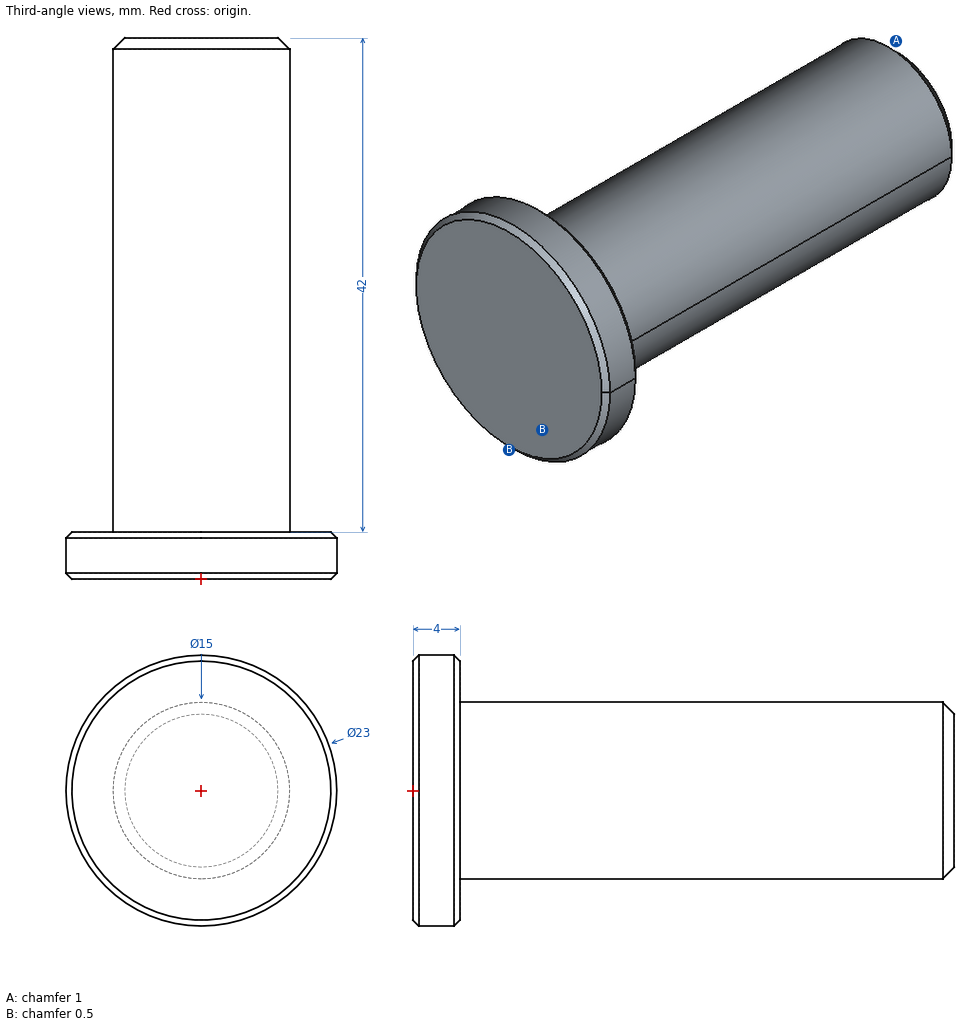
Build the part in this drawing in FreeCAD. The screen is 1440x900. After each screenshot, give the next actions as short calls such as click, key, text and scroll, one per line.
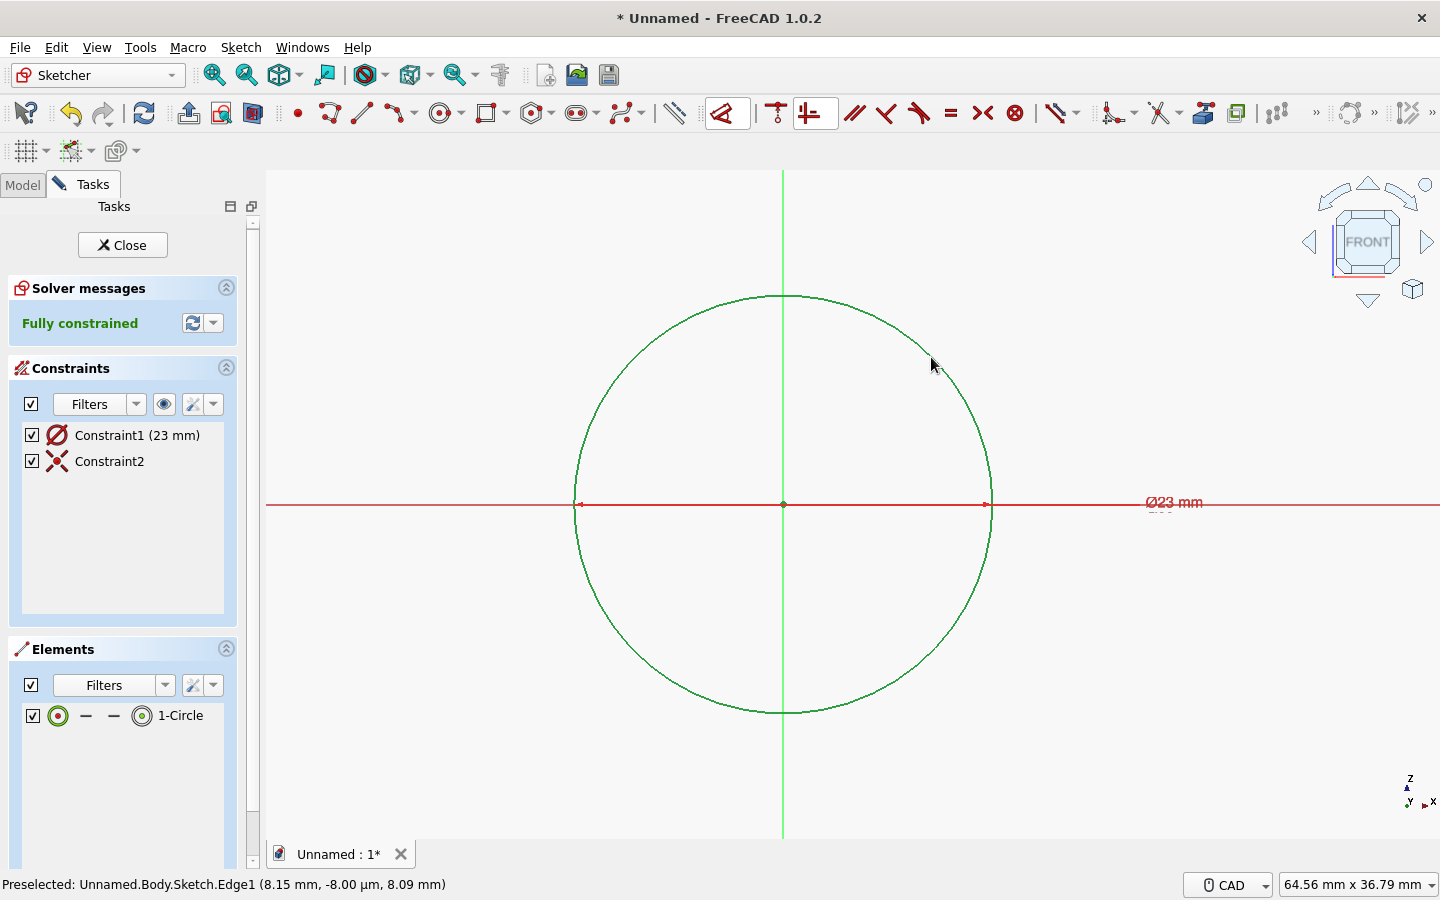
click(123, 245)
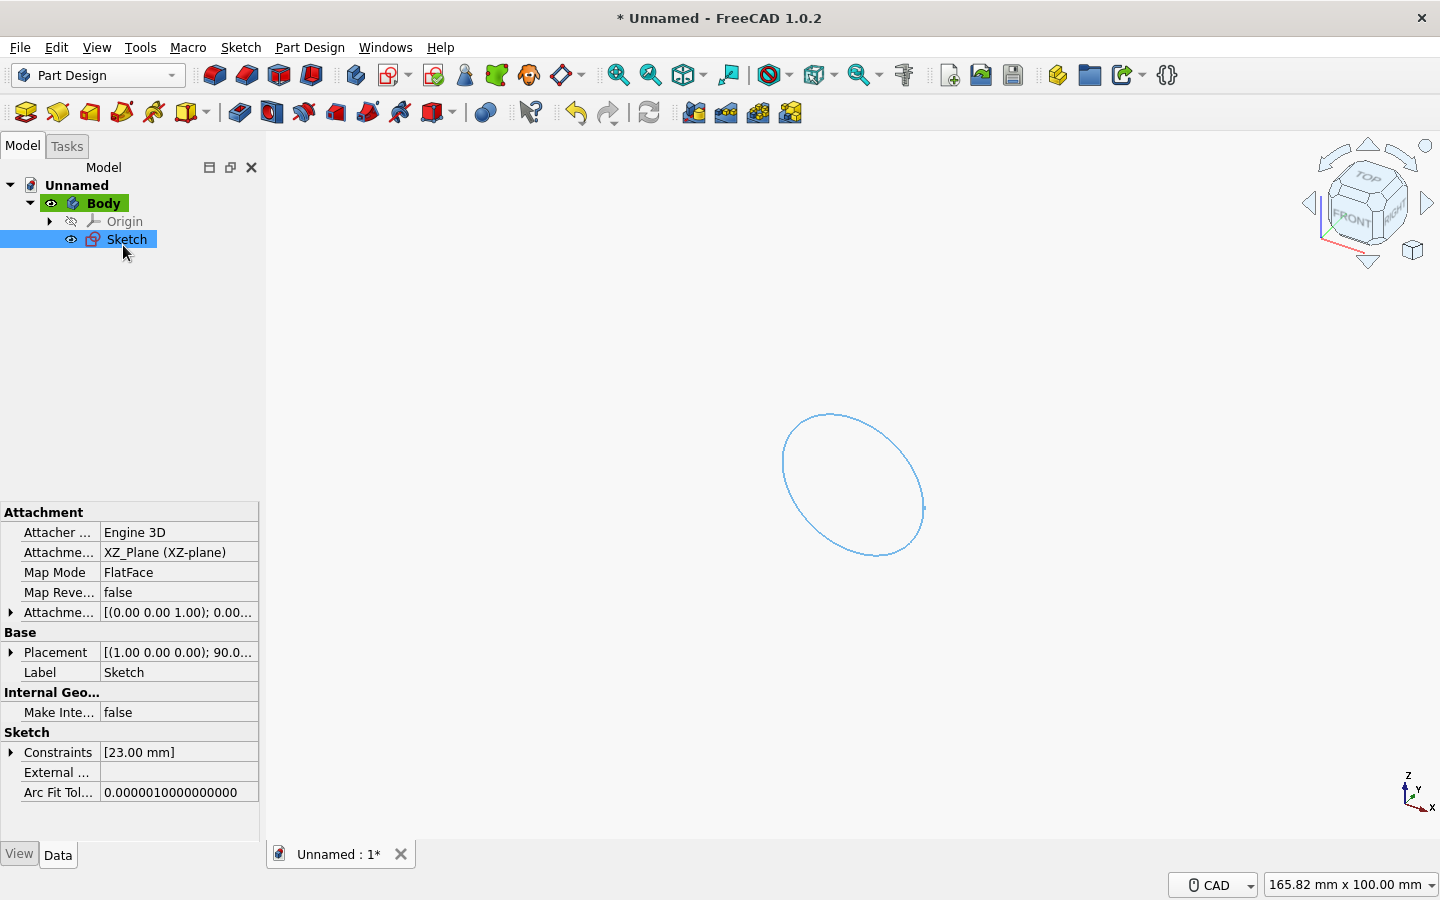
click(26, 112)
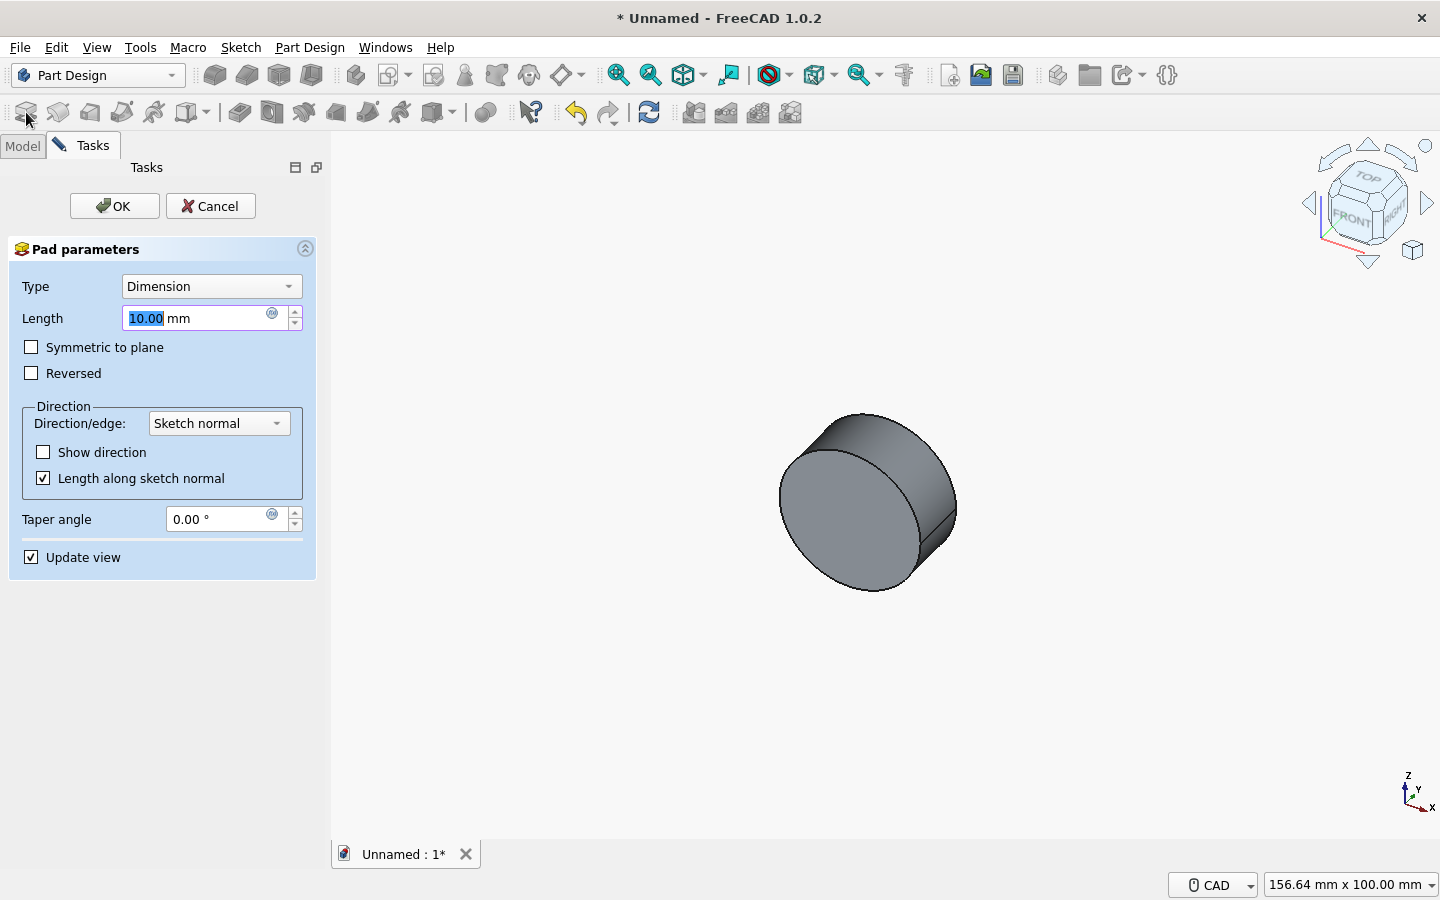
text(4)
key(Tab)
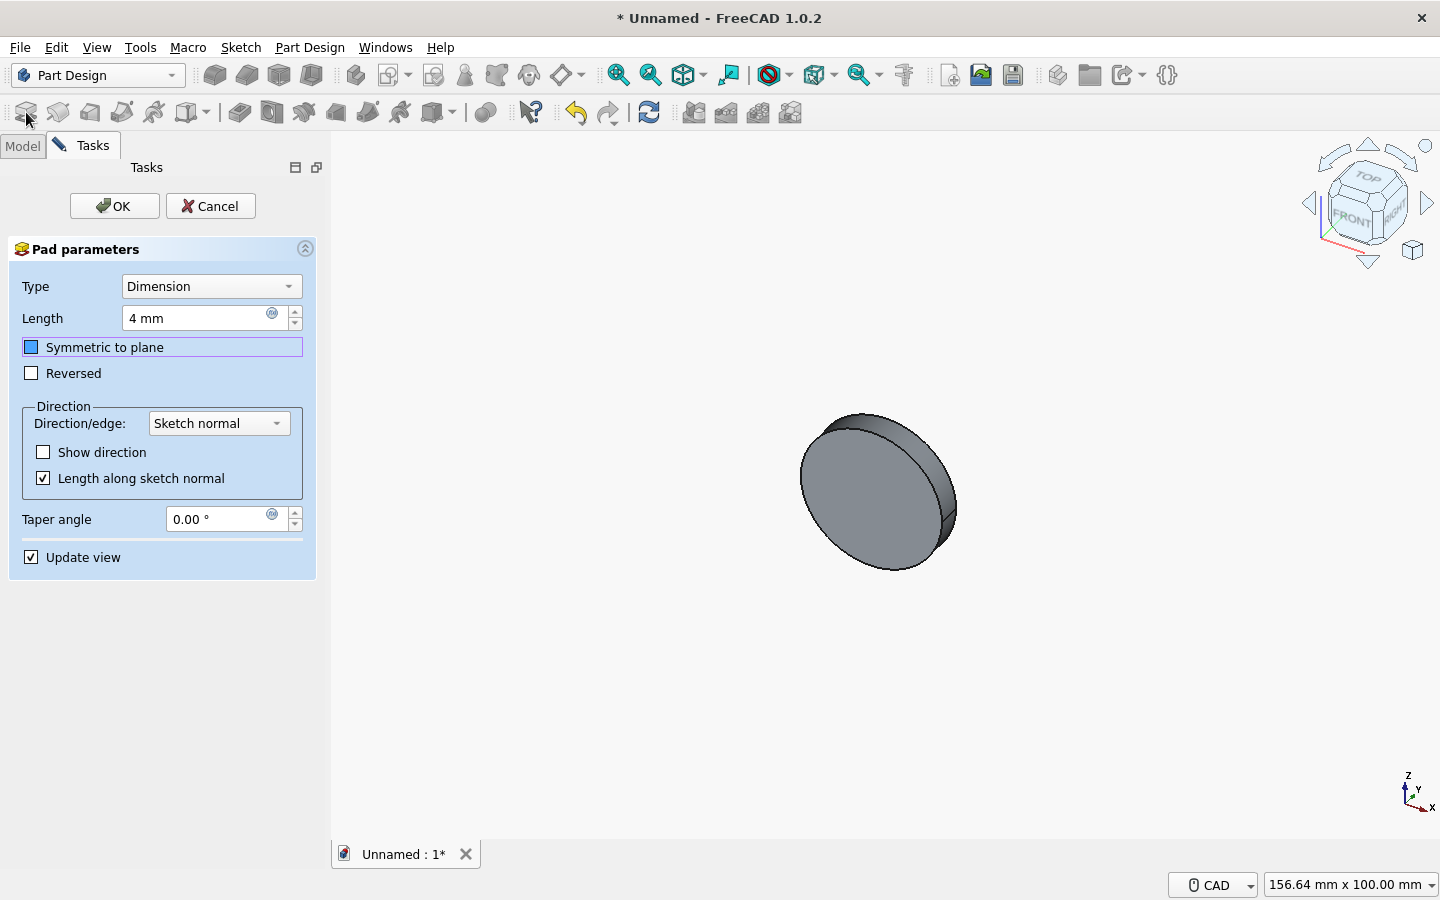
click(30, 373)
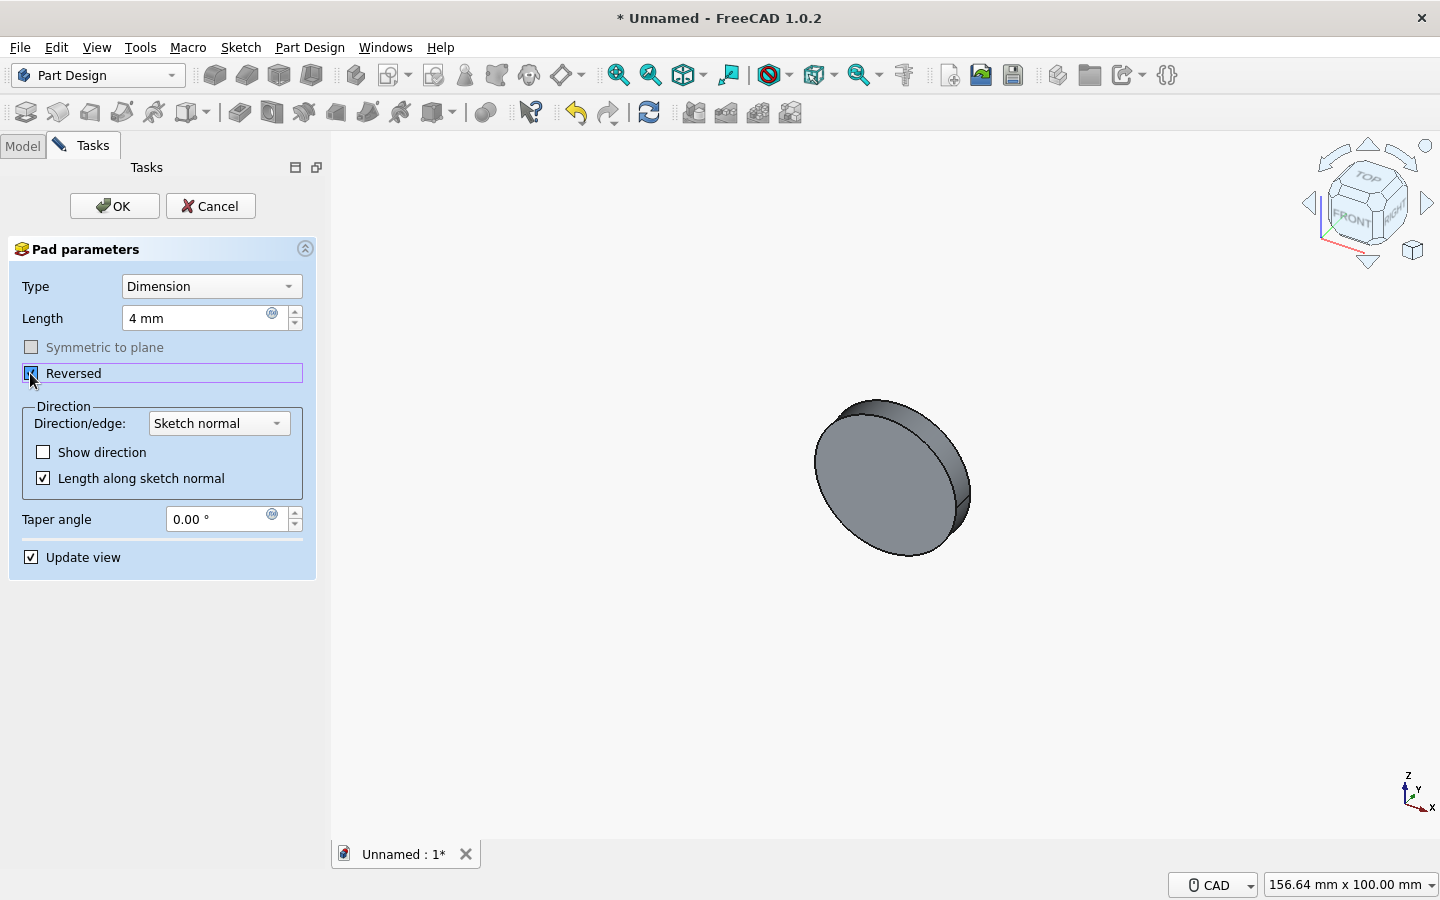
click(115, 206)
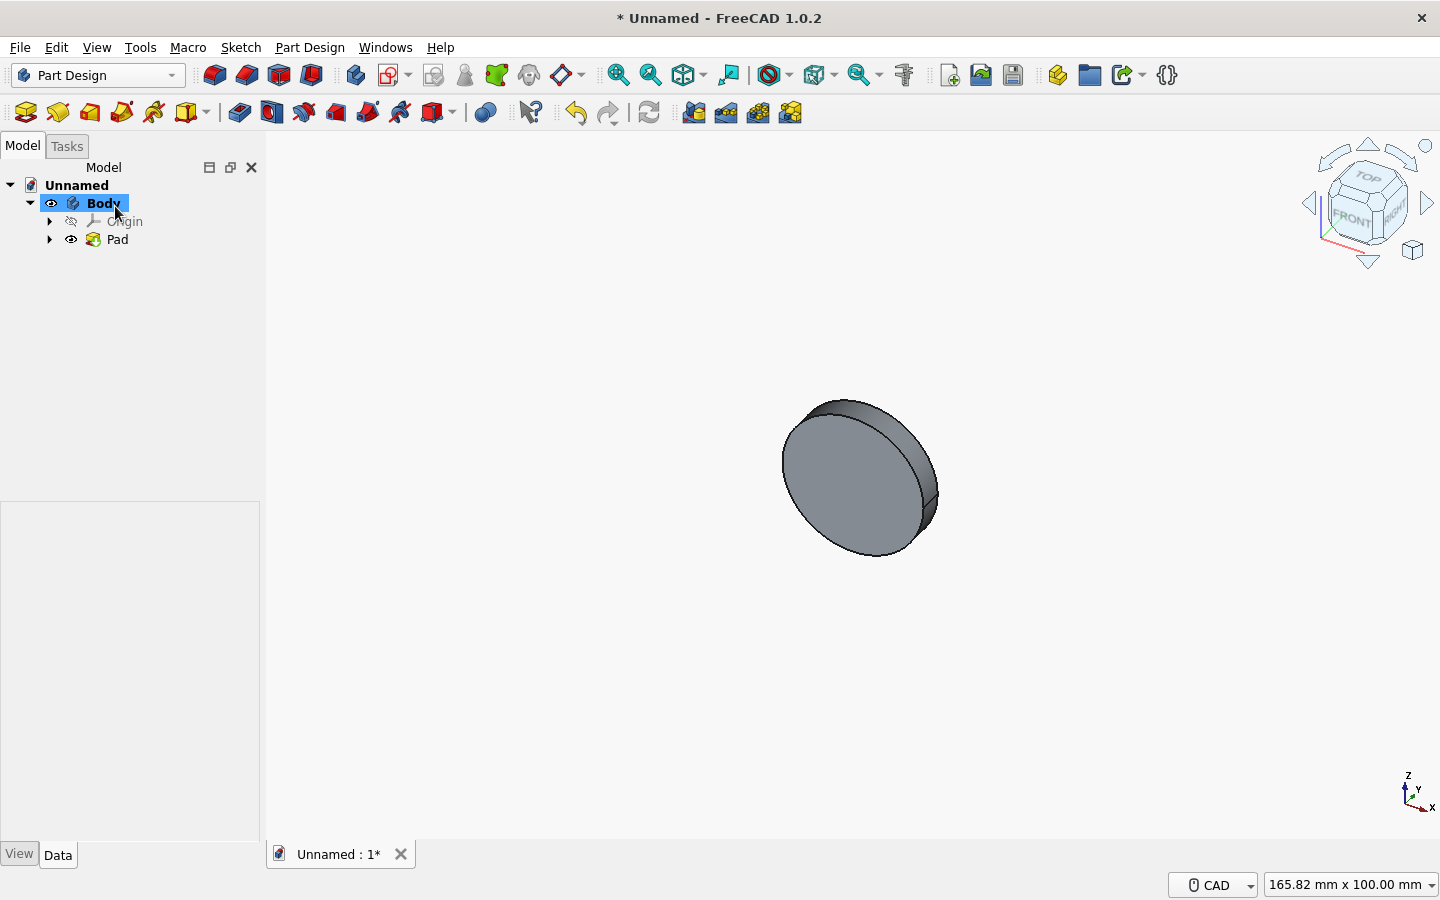
click(620, 76)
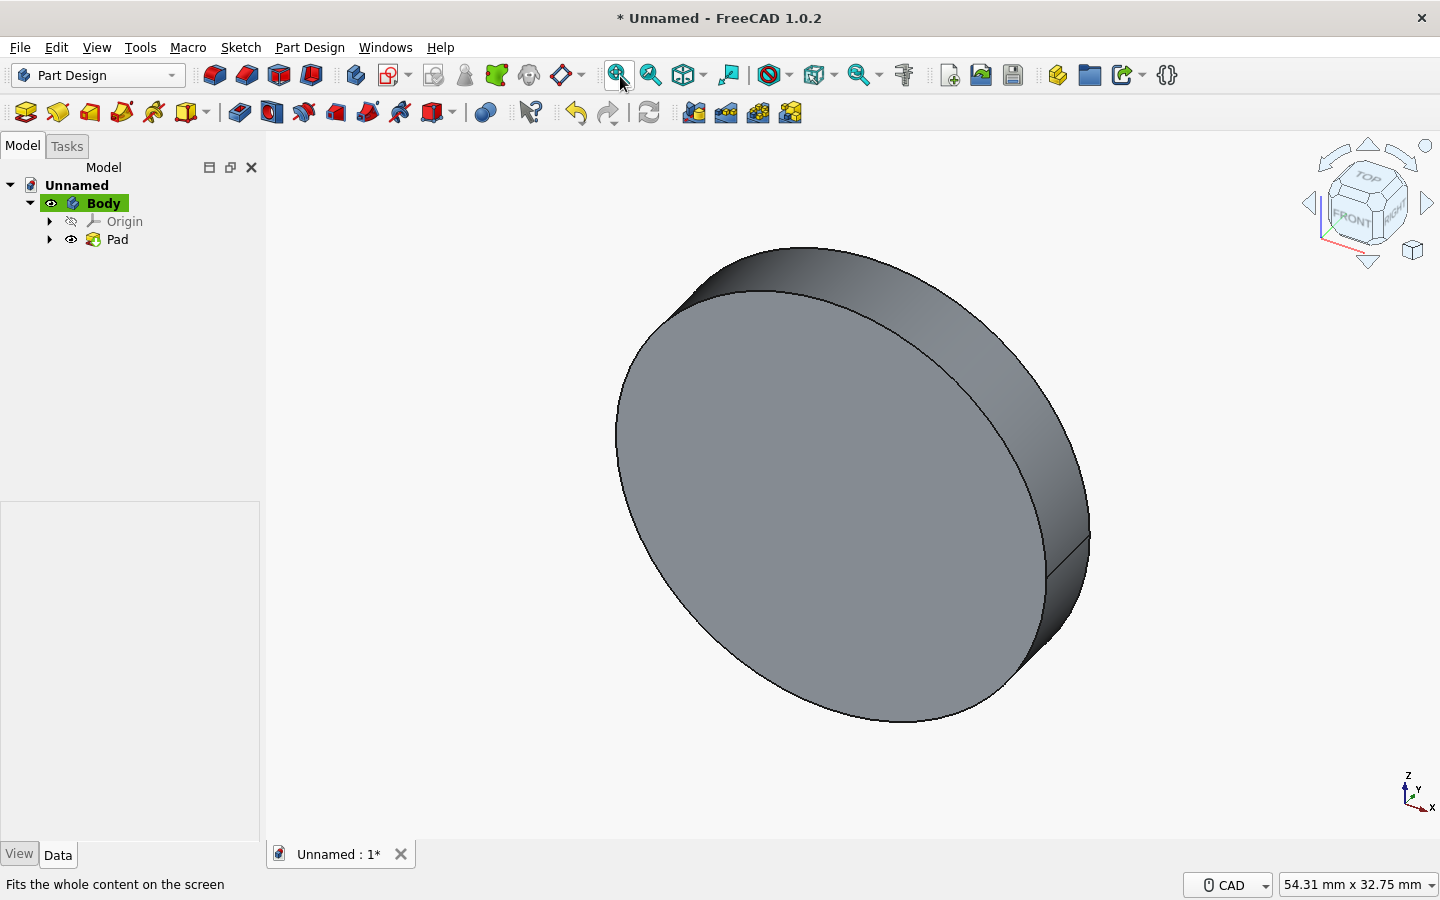
key(4)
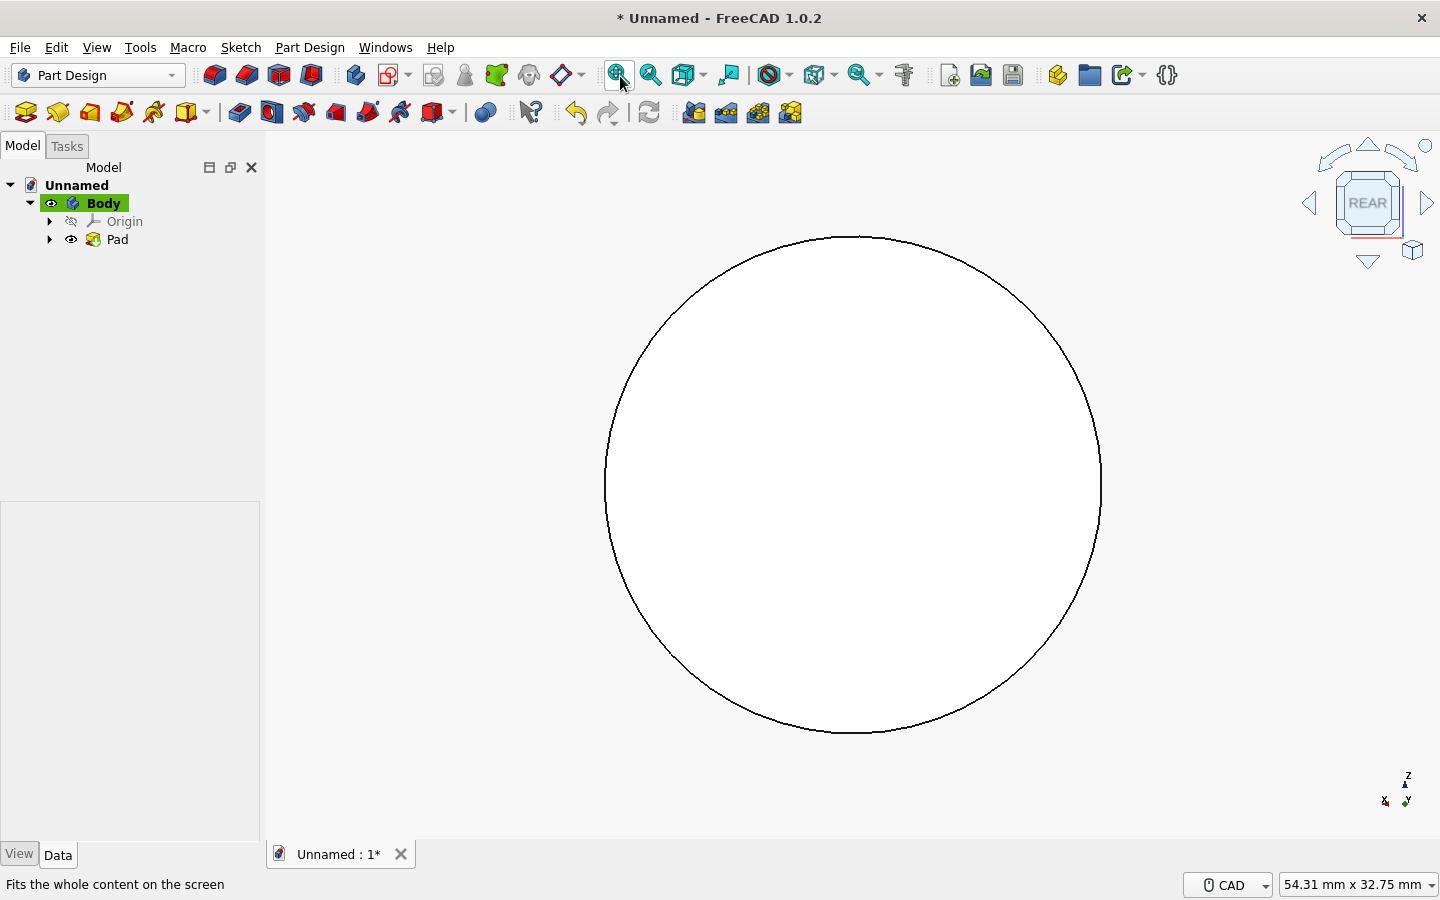
click(853, 484)